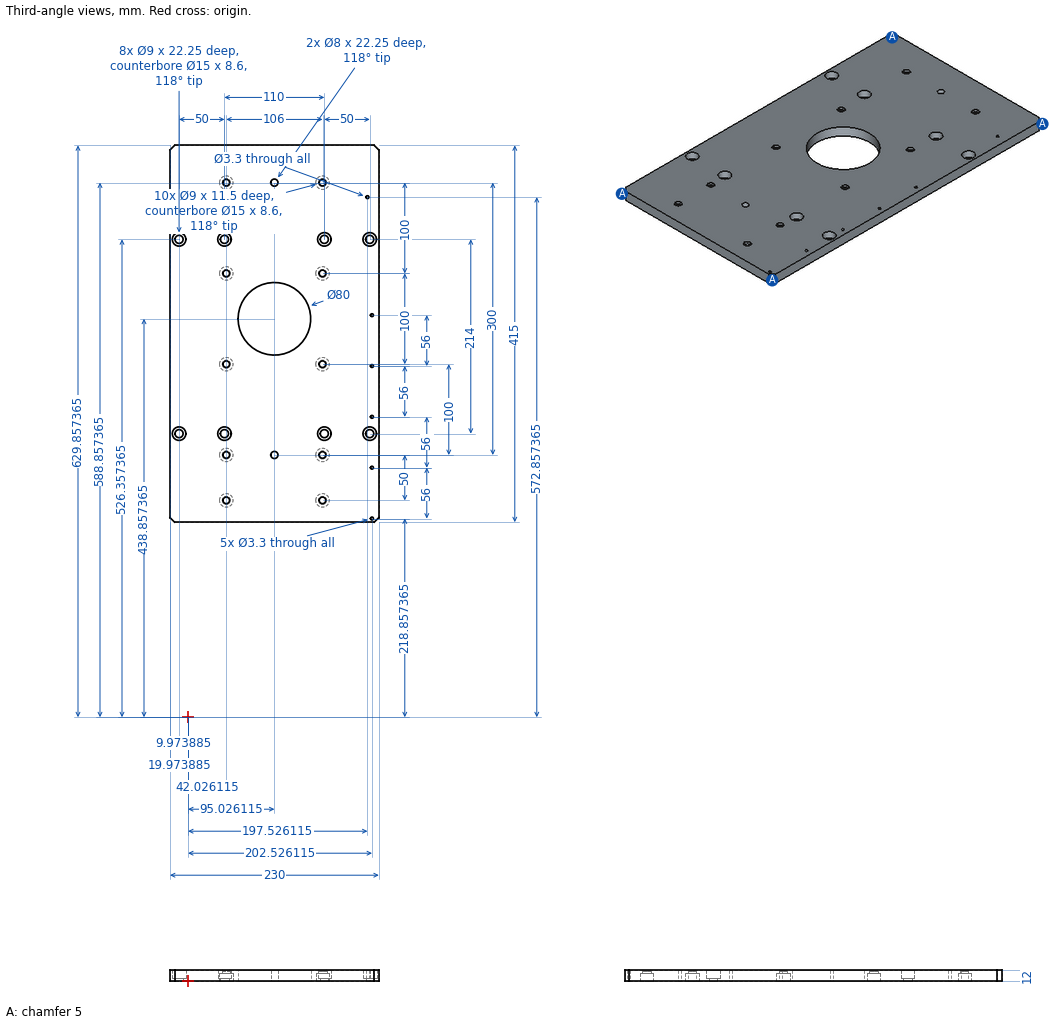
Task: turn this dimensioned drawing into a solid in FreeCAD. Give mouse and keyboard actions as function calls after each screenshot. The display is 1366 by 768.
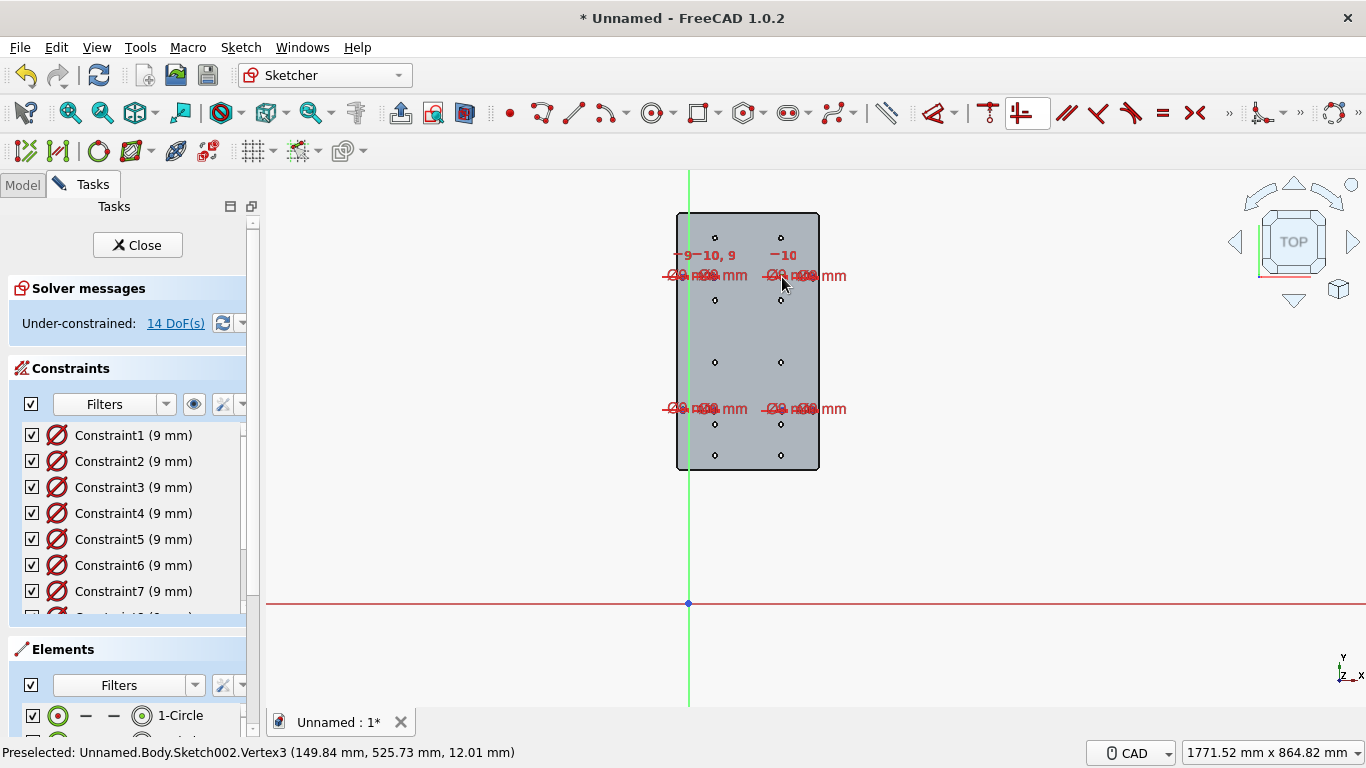
click(813, 278)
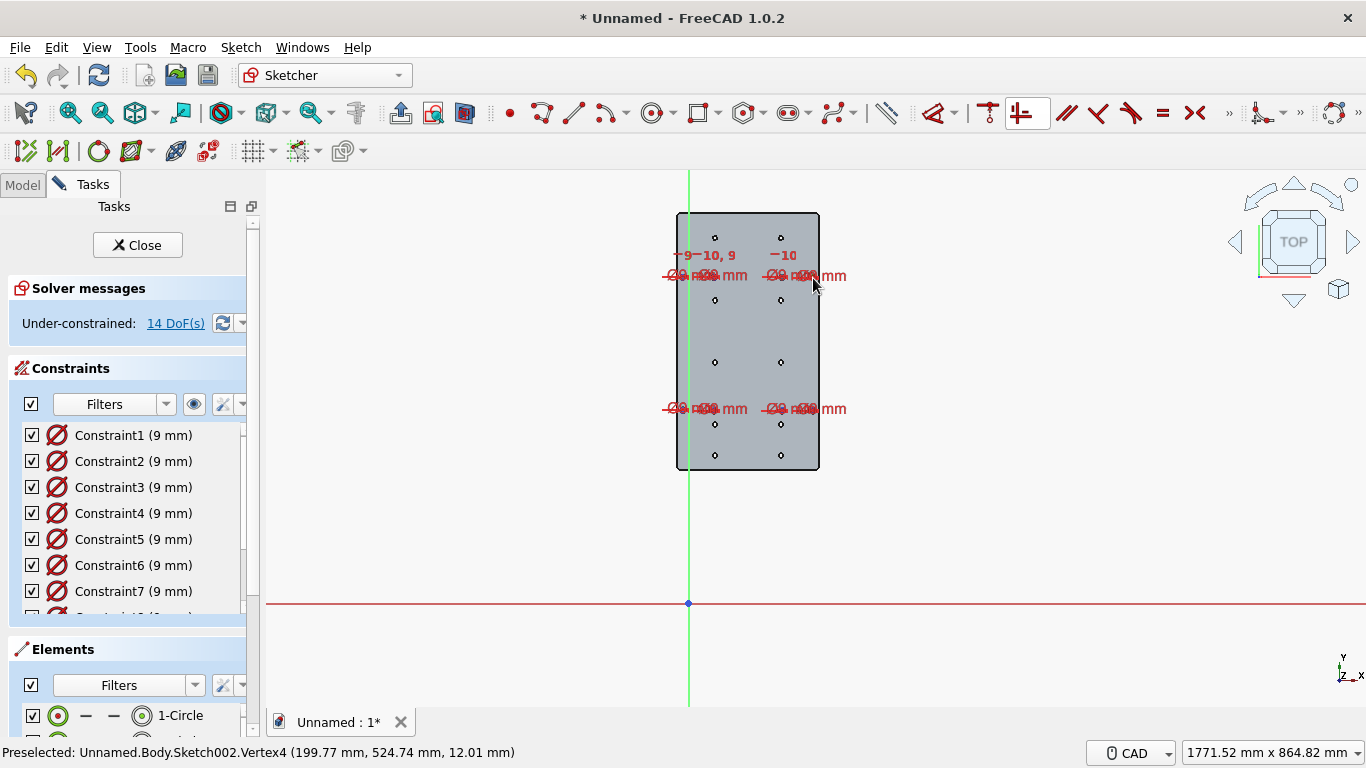
click(1044, 114)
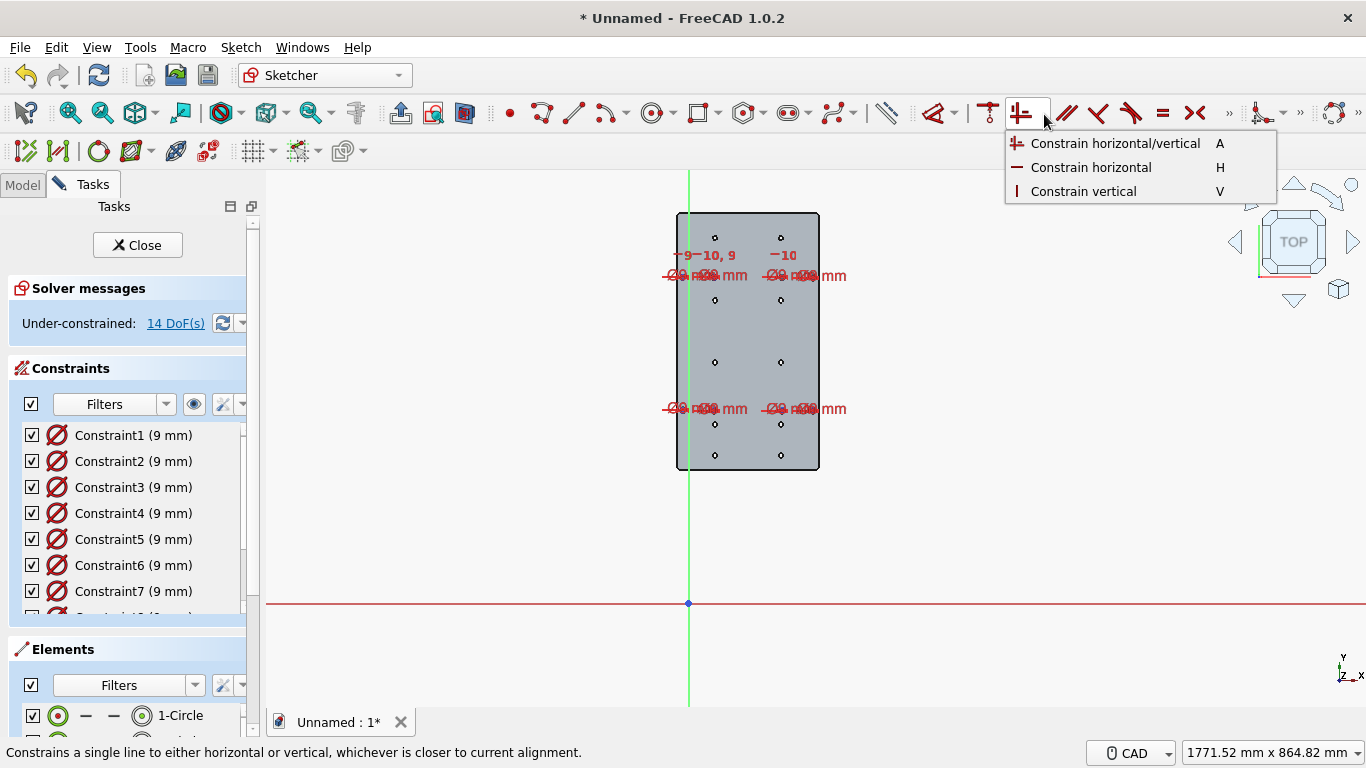
click(1141, 167)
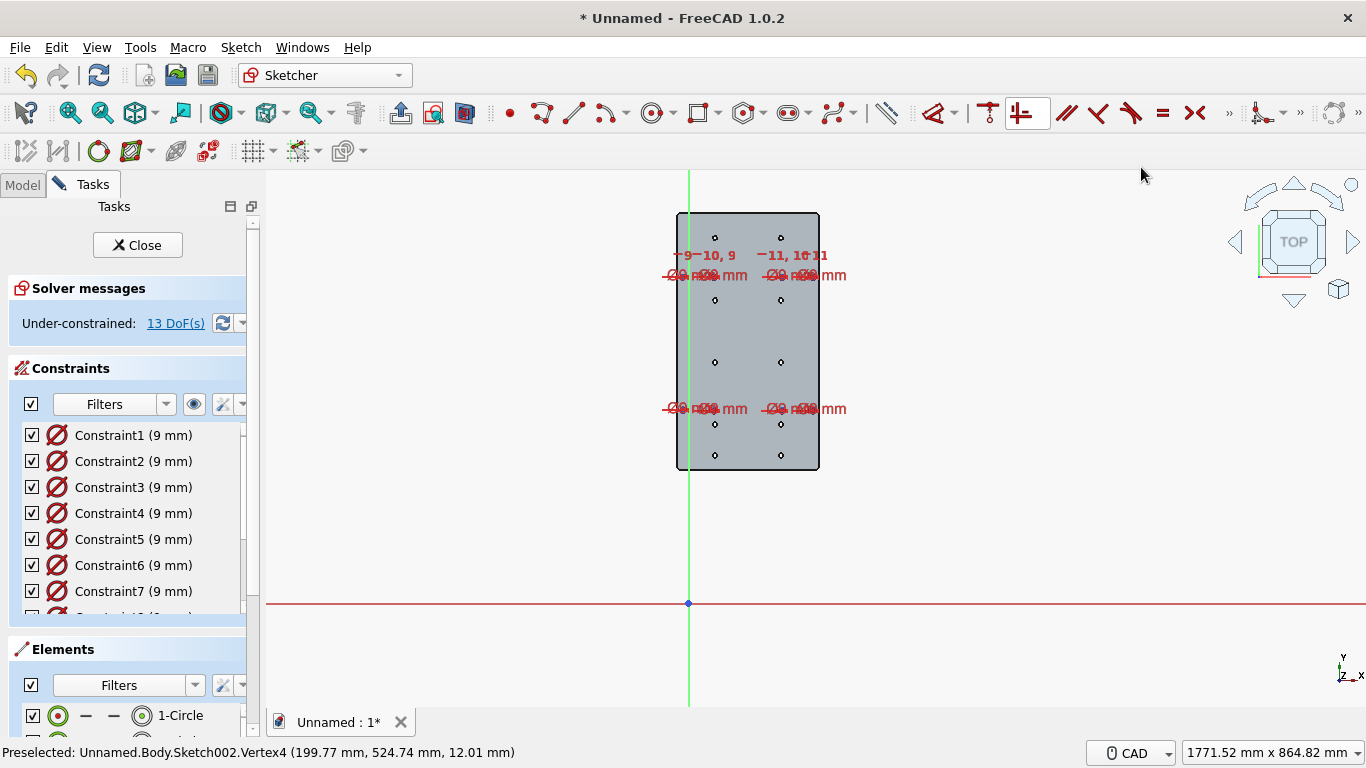
click(813, 277)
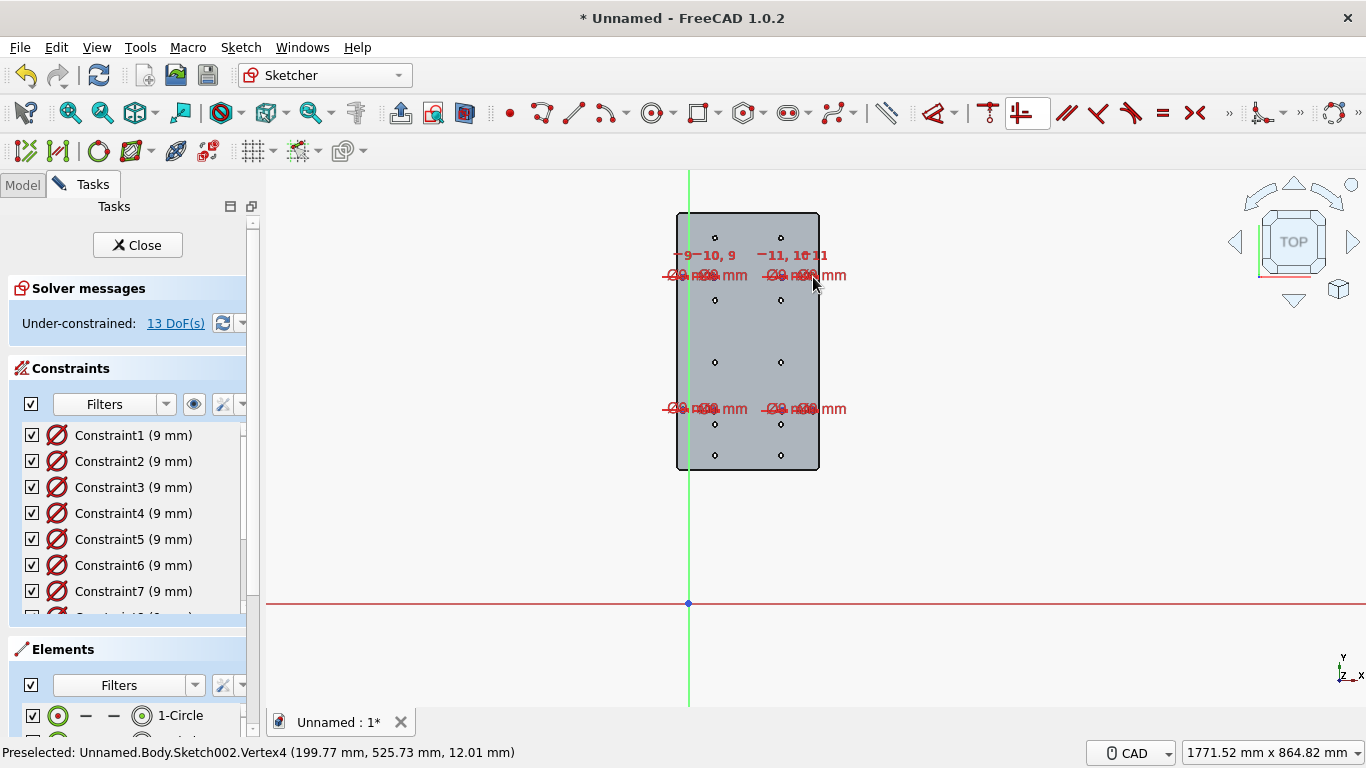
click(813, 411)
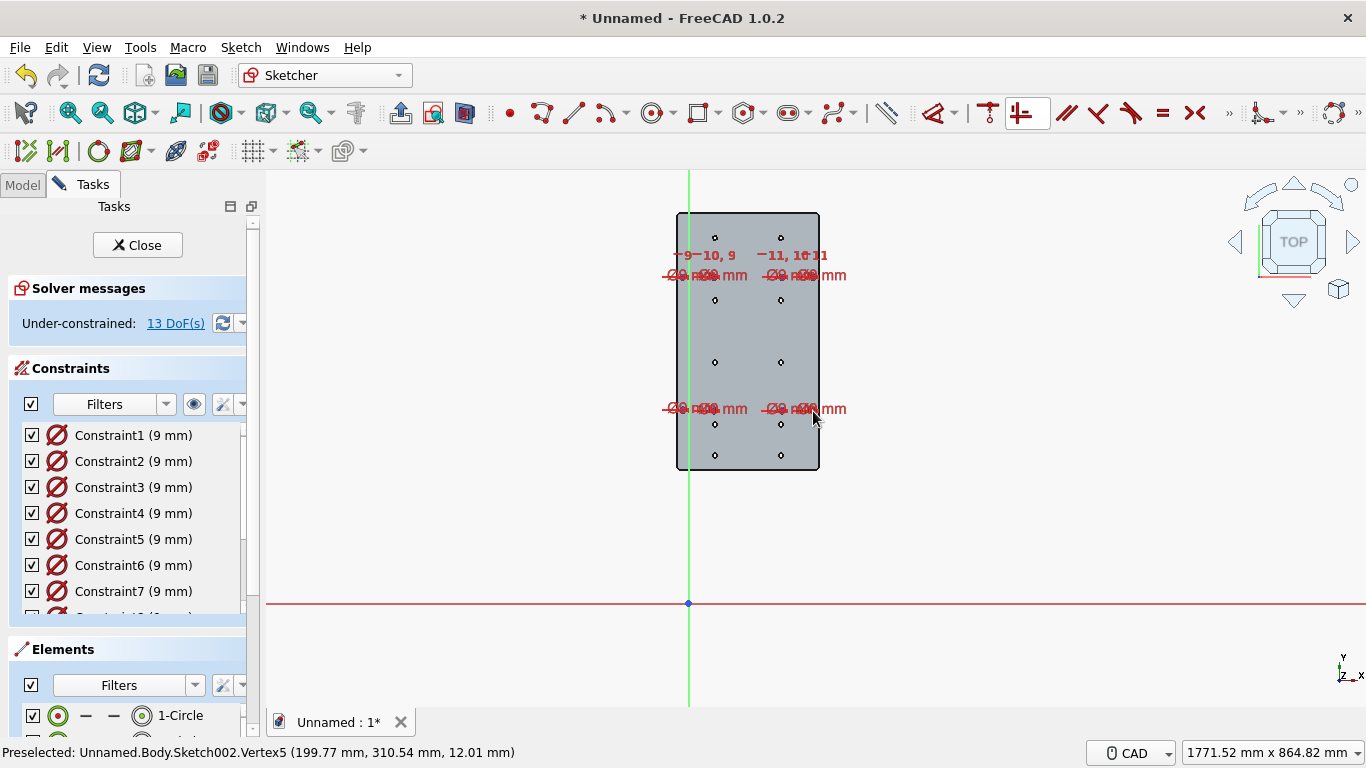
click(1044, 114)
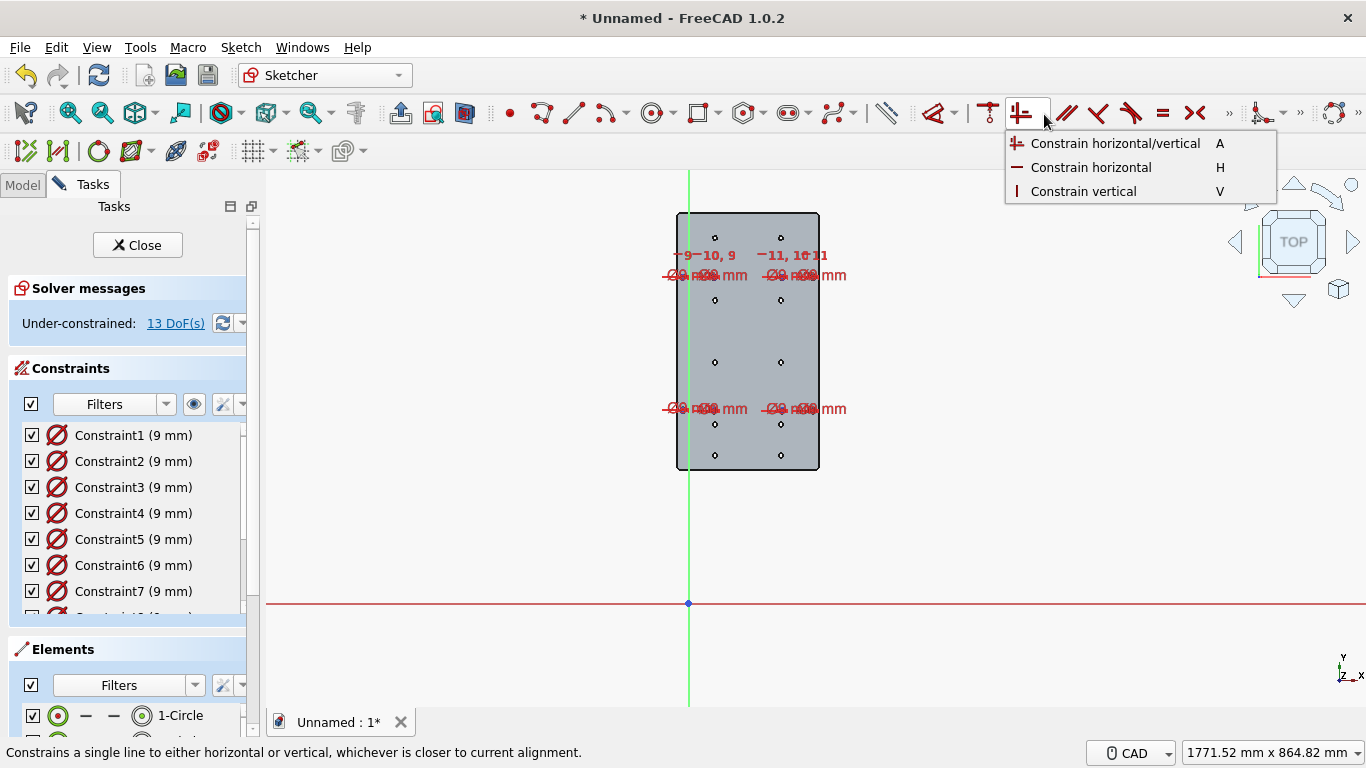
click(1141, 191)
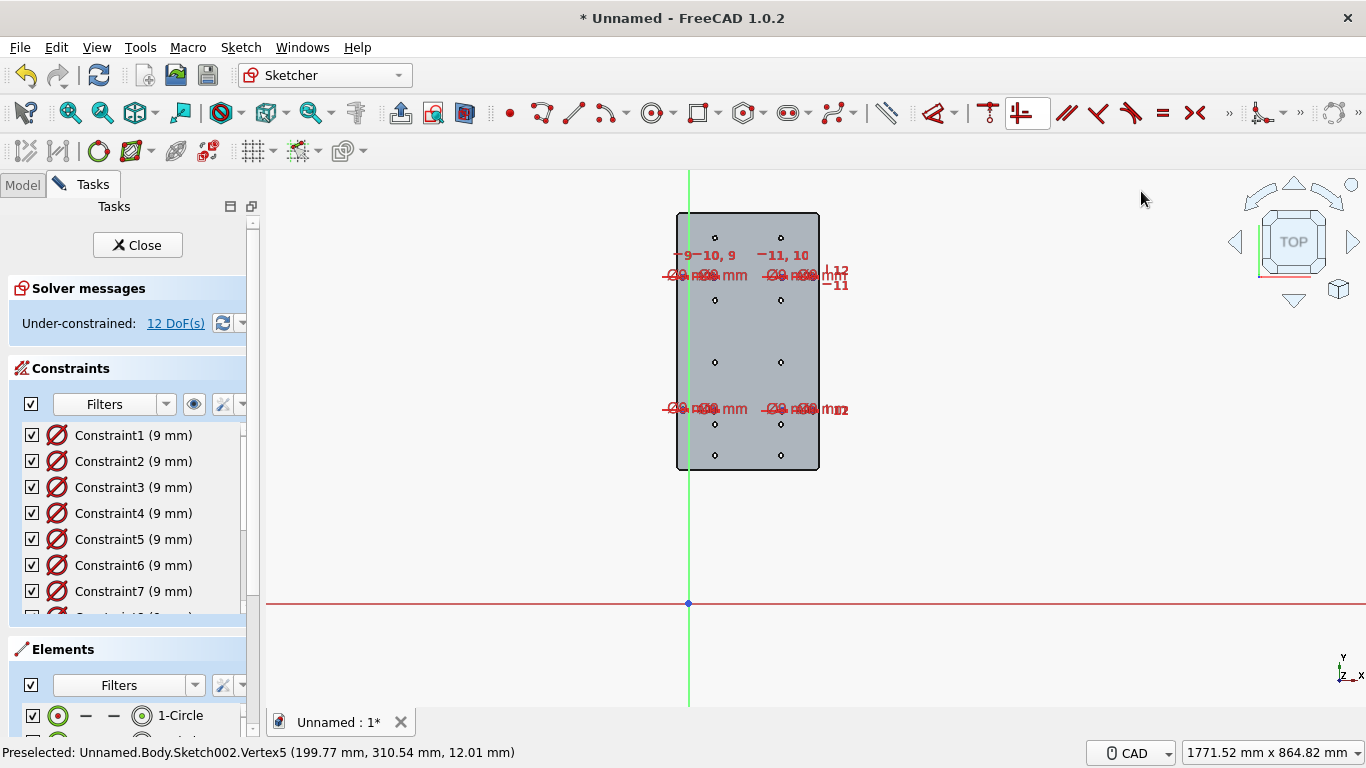
click(782, 277)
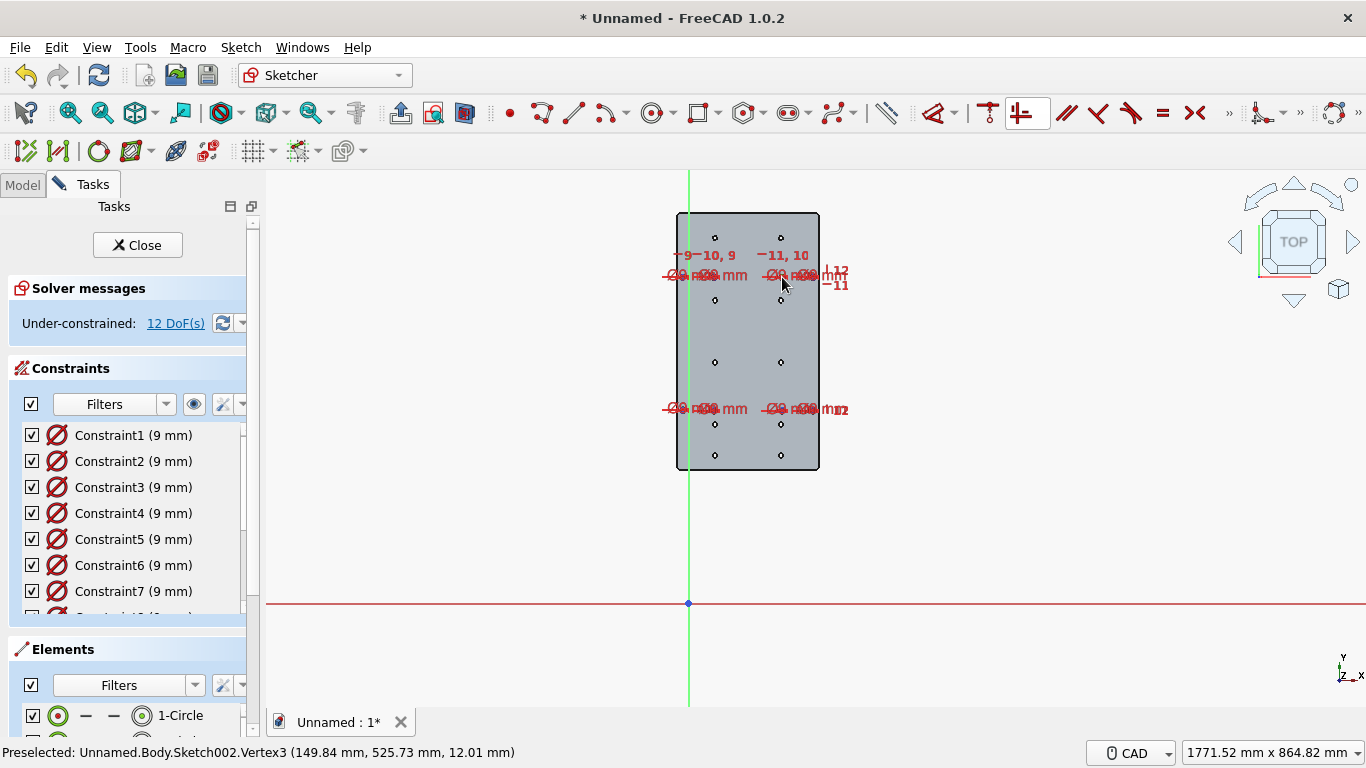
click(782, 411)